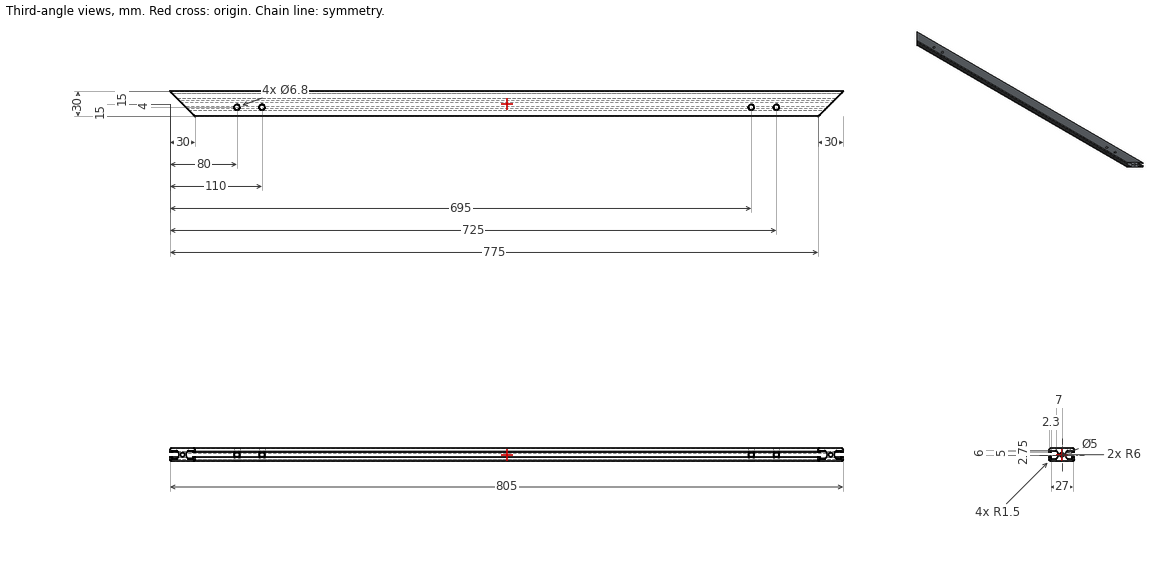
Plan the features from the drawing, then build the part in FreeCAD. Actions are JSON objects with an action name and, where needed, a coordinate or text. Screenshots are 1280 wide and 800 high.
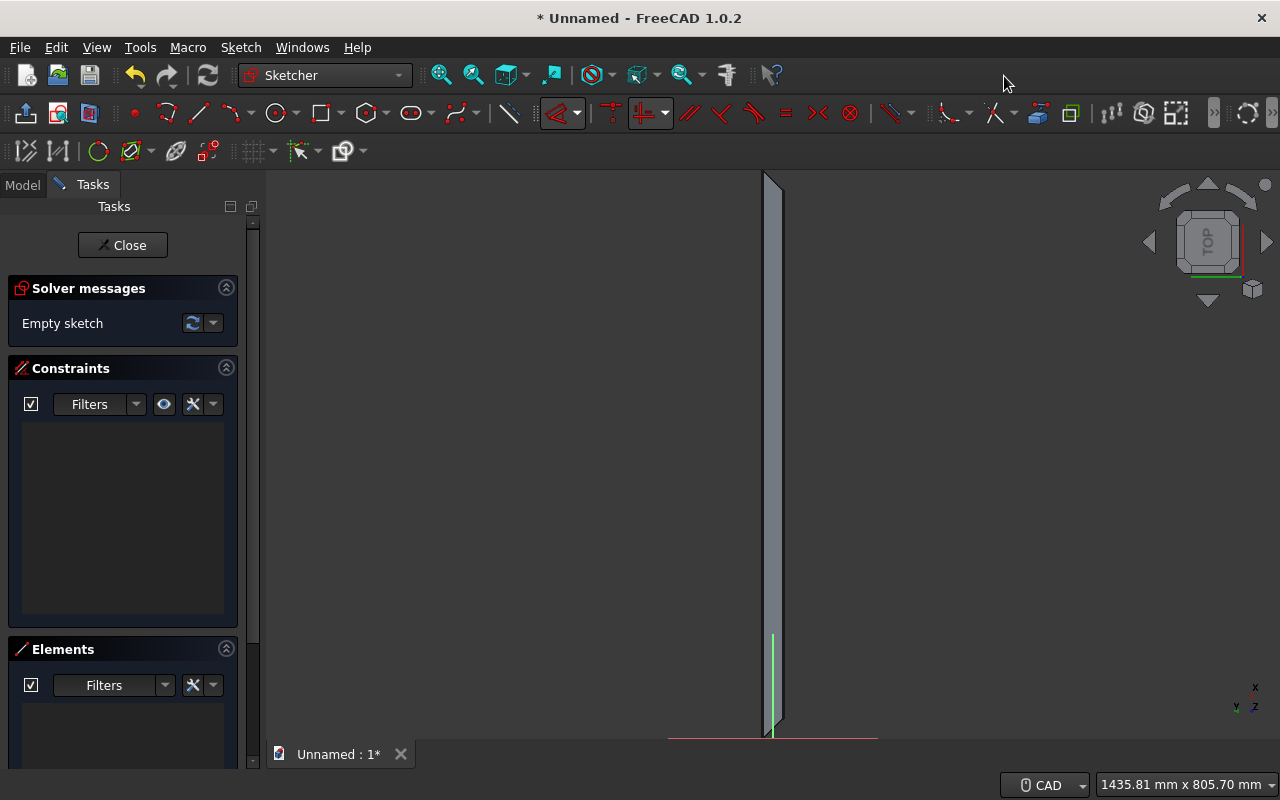
{"action": "scroll", "coordinate": [560, 400], "scroll_direction": "down", "scroll_amount": 2}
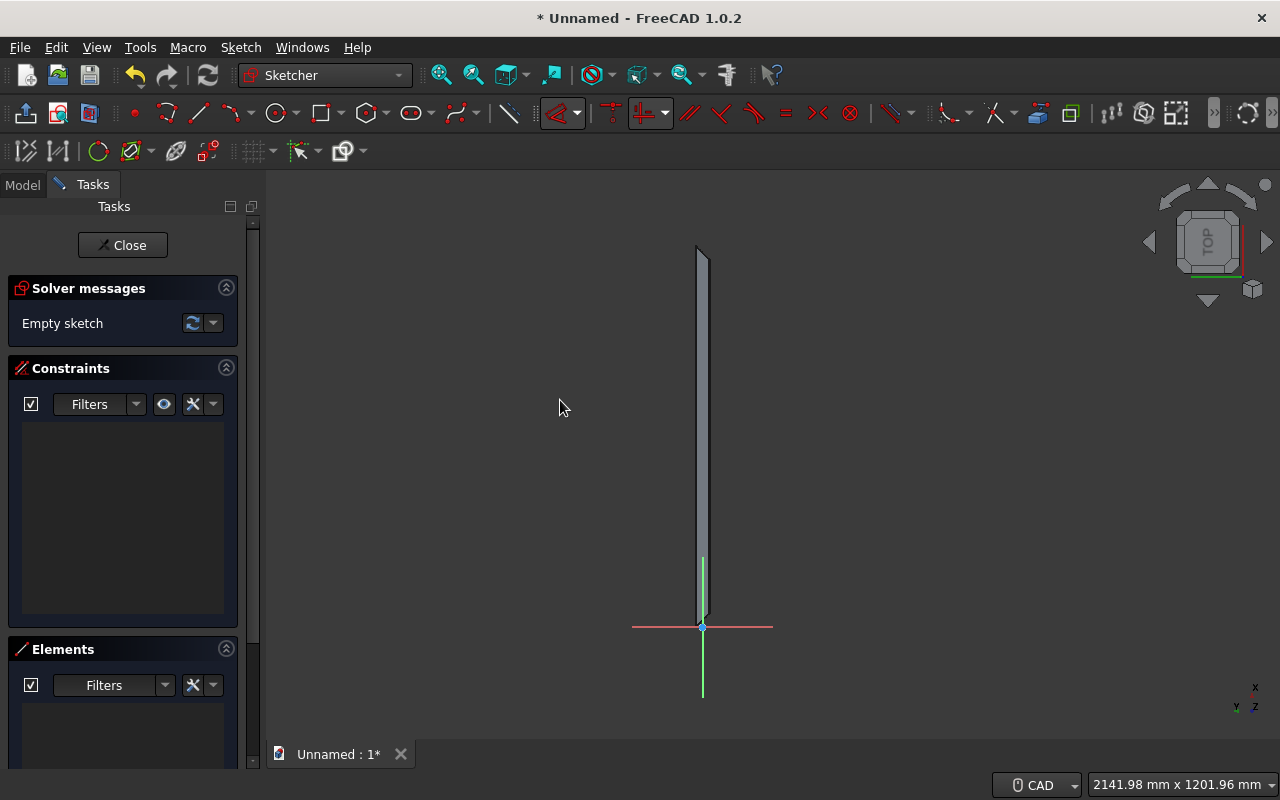
{"action": "left_click", "coordinate": [276, 114]}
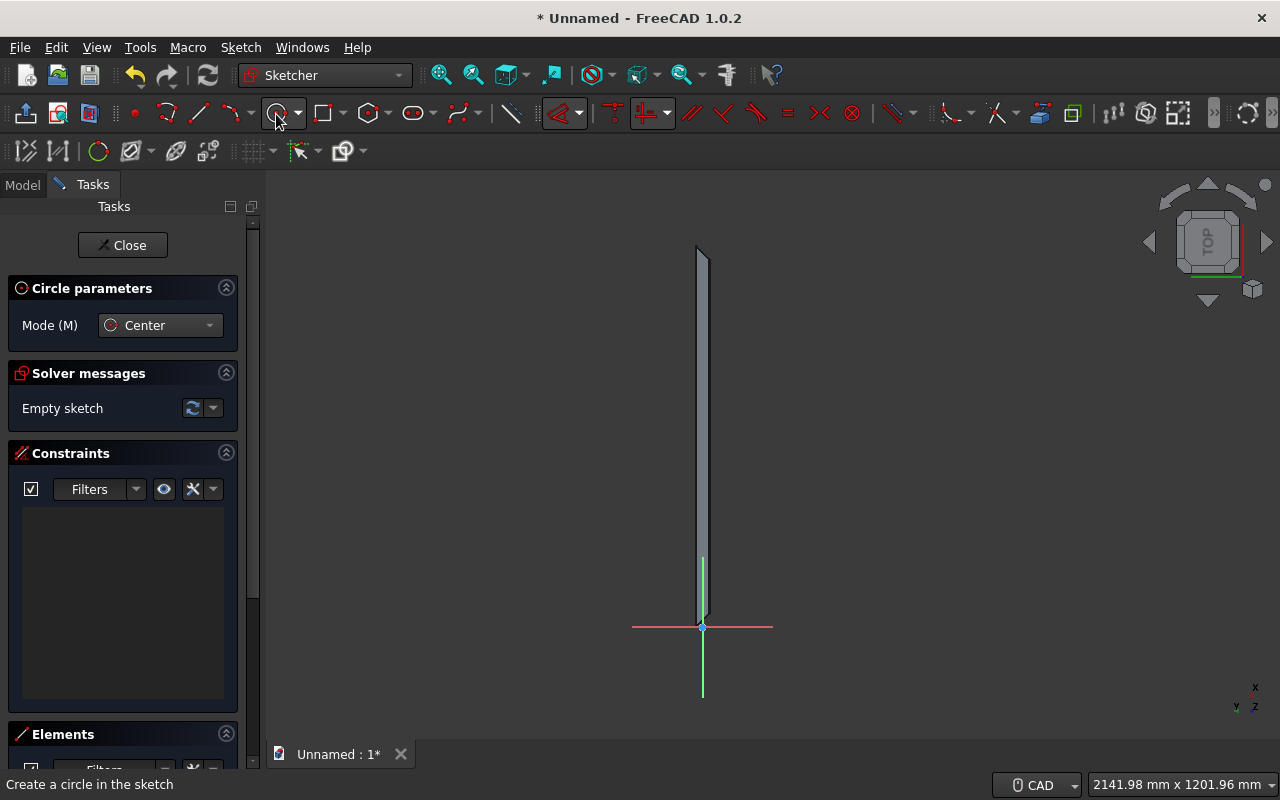
{"action": "scroll", "coordinate": [705, 589], "scroll_direction": "up", "scroll_amount": 14}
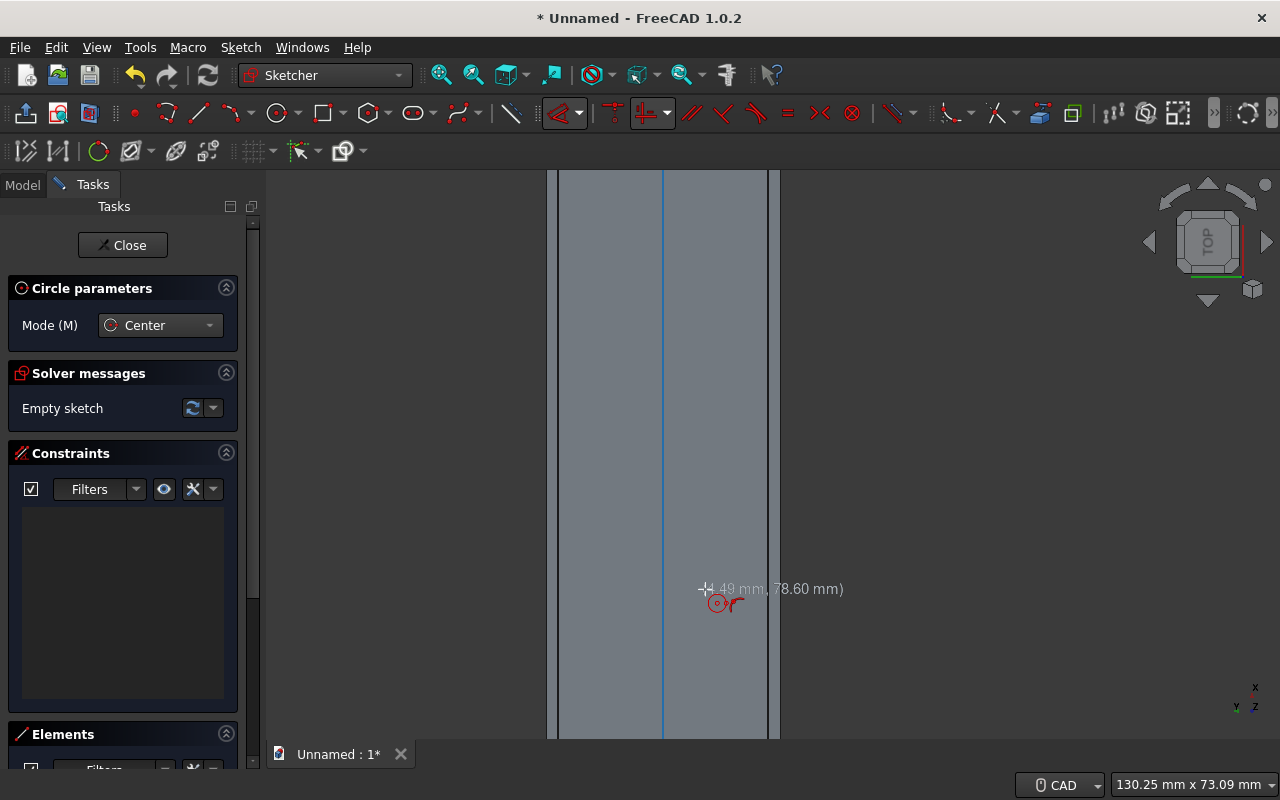
{"action": "left_click", "coordinate": [694, 583]}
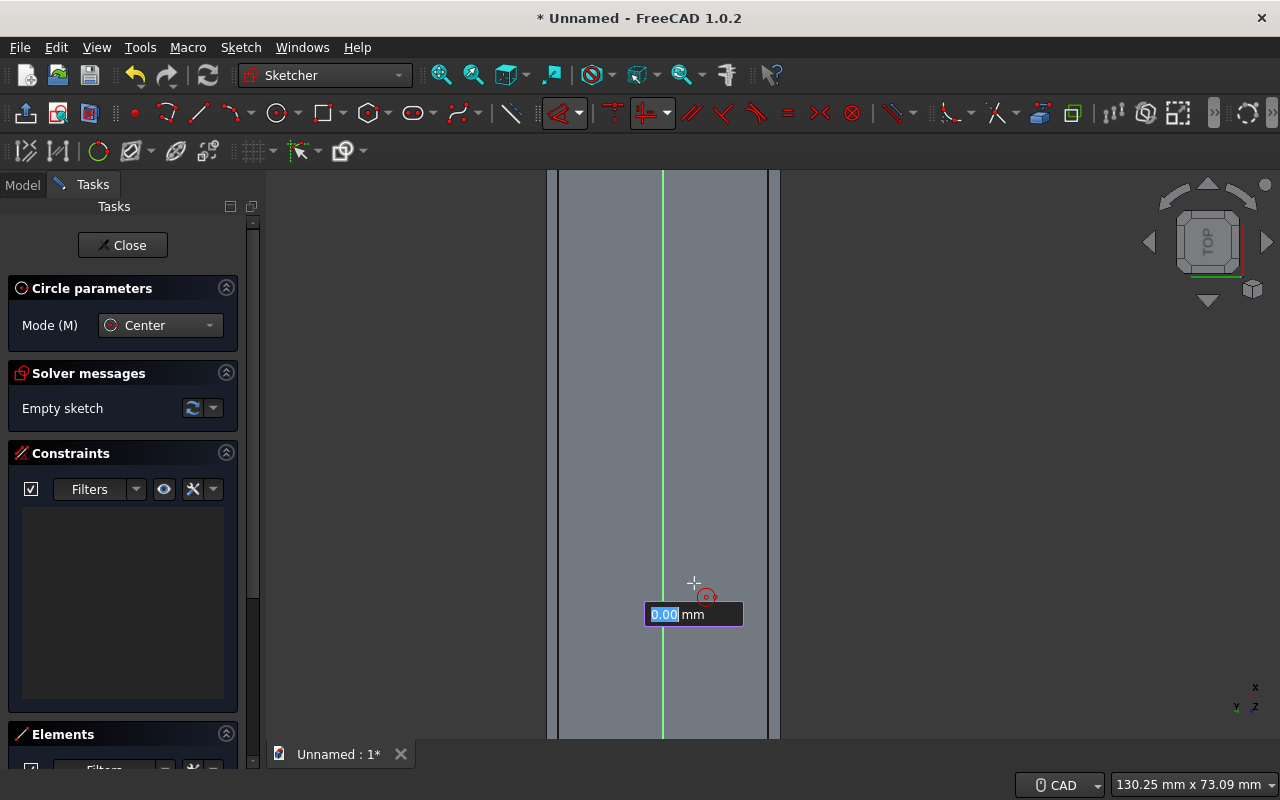
{"action": "scroll", "coordinate": [705, 589], "scroll_direction": "down", "scroll_amount": 14}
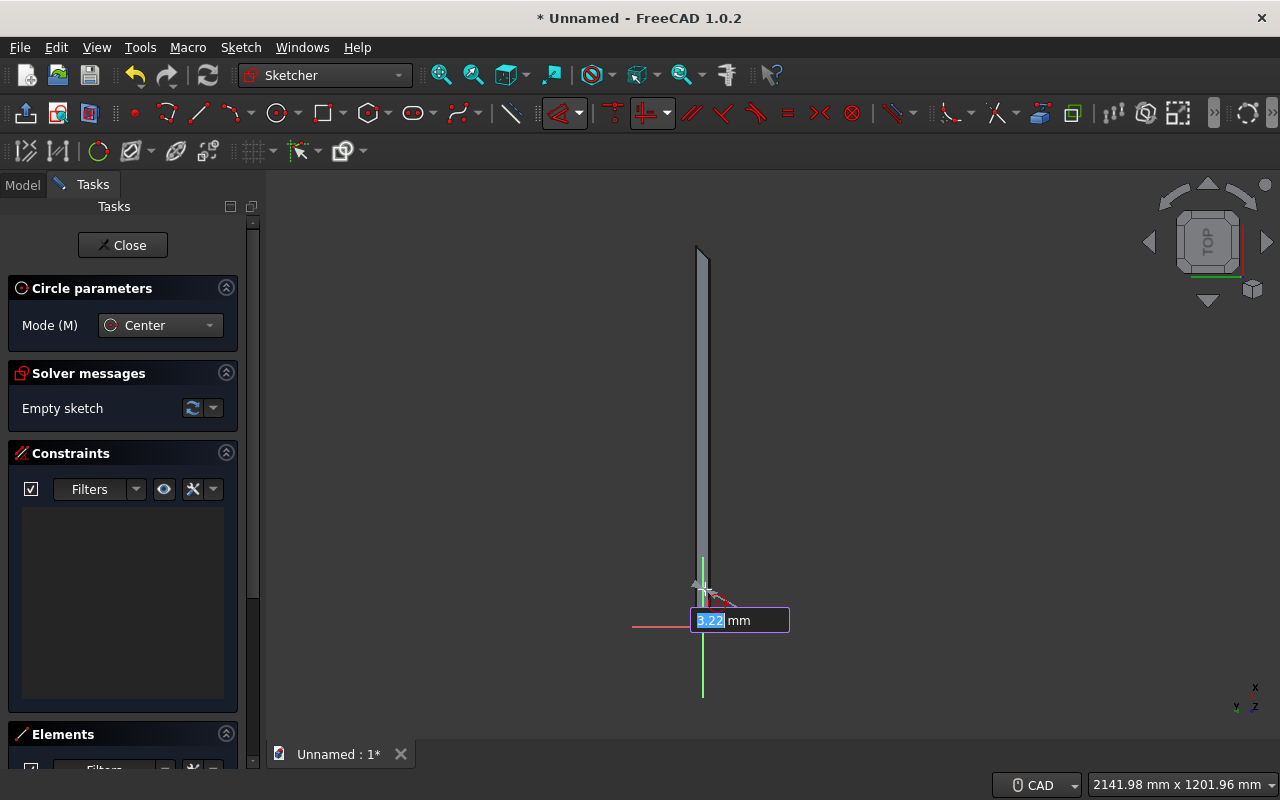
{"action": "scroll", "coordinate": [706, 588], "scroll_direction": "up", "scroll_amount": 9}
{"action": "mouse_move", "coordinate": [703, 585]}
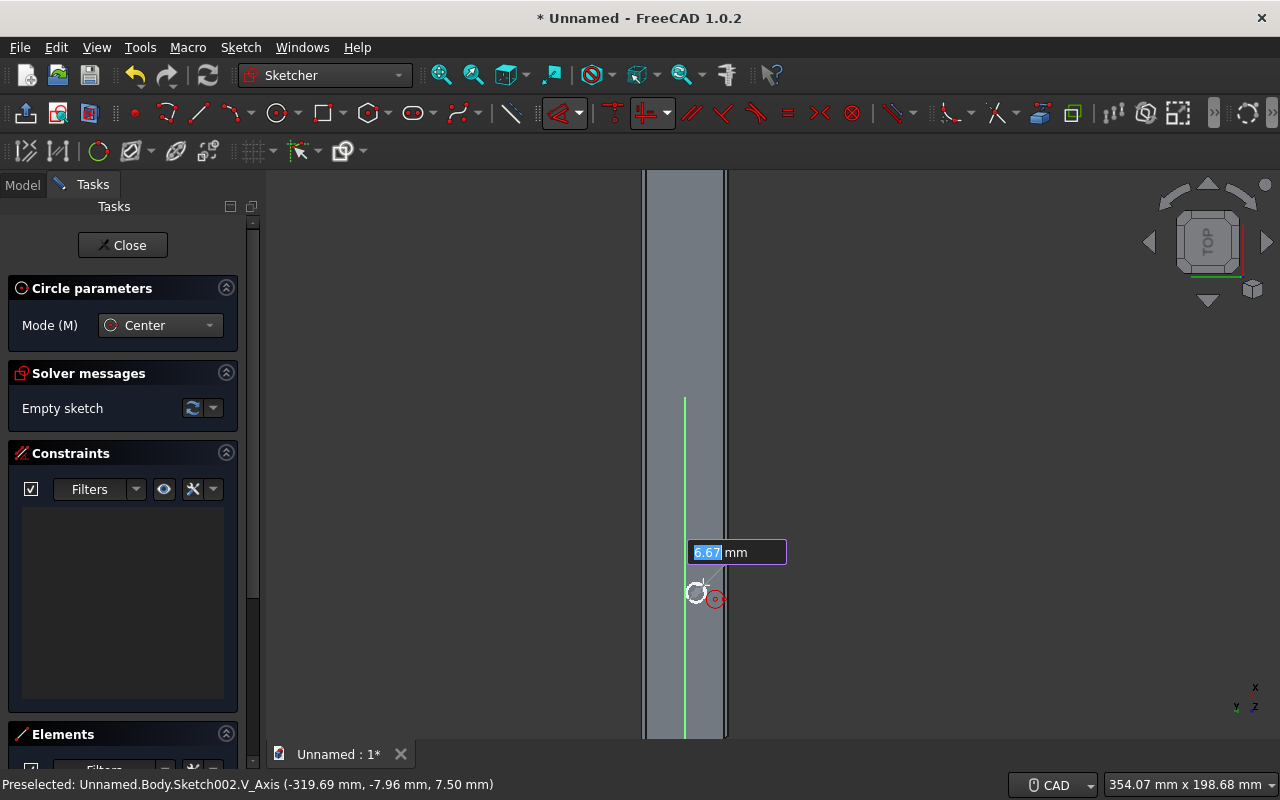
{"action": "type", "text": "6.8"}
{"action": "key", "text": "Return"}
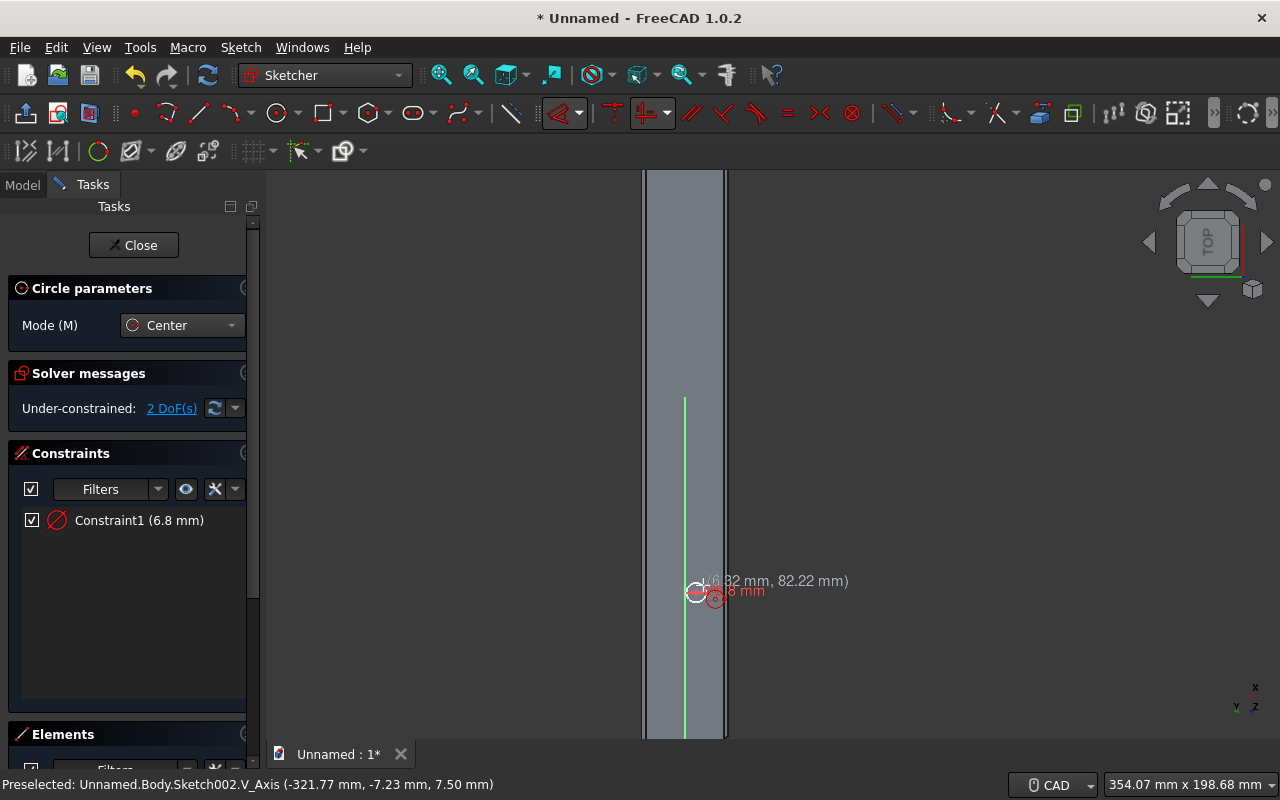
{"action": "scroll", "coordinate": [696, 506], "scroll_direction": "up", "scroll_amount": 5}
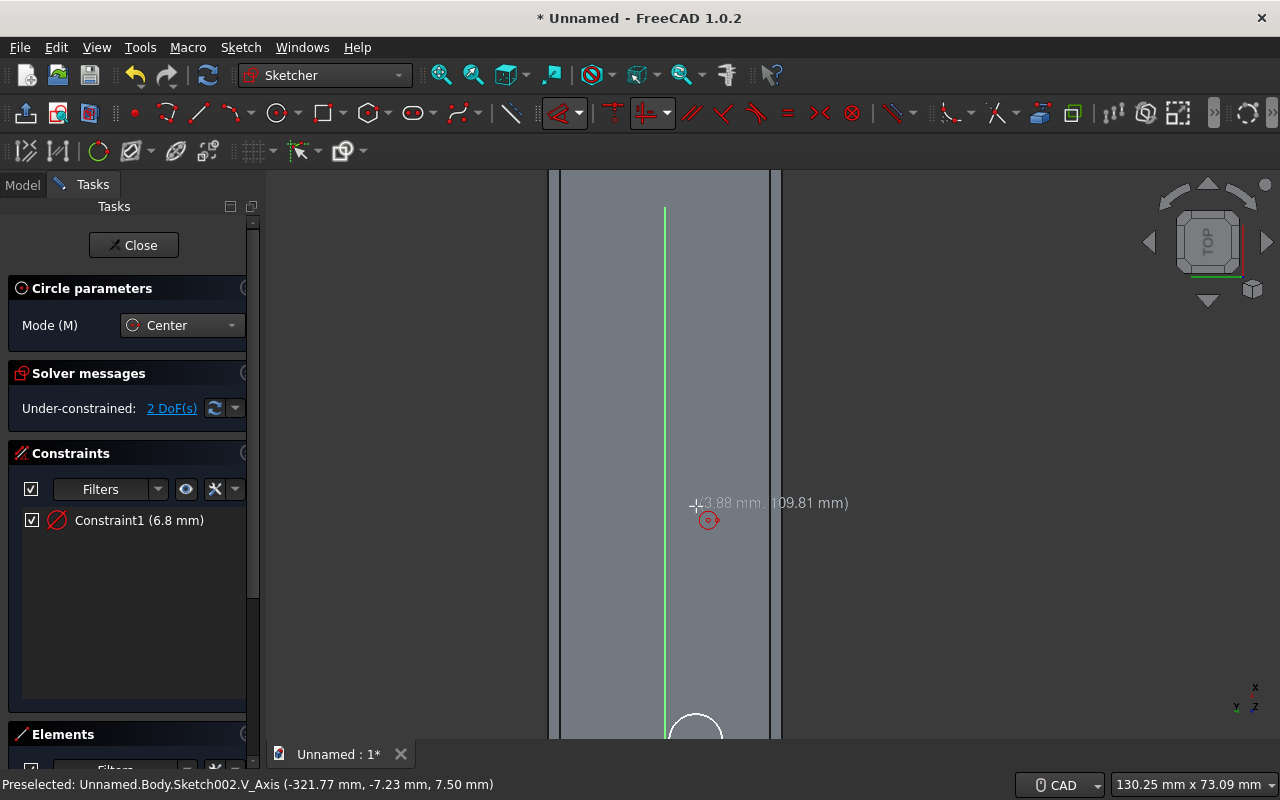
{"action": "left_click", "coordinate": [696, 506]}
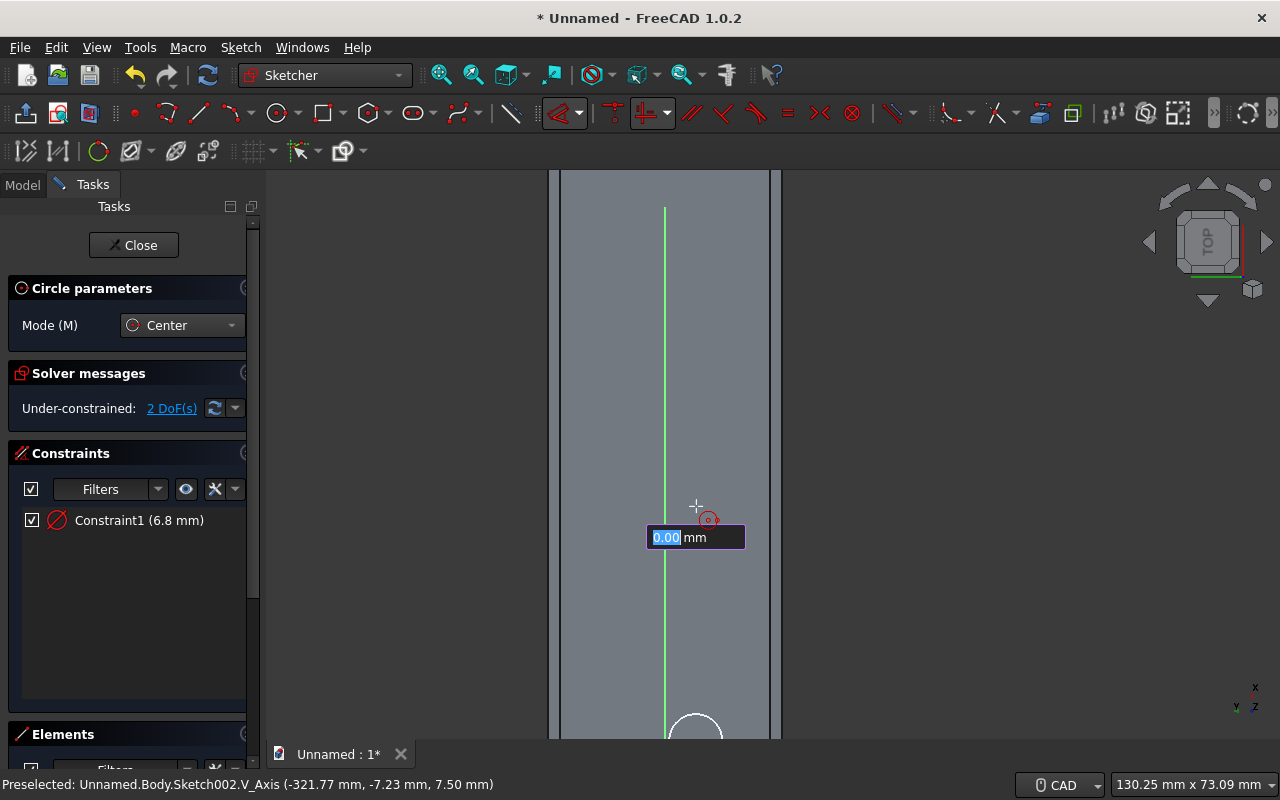
{"action": "scroll", "coordinate": [705, 579], "scroll_direction": "down", "scroll_amount": 14}